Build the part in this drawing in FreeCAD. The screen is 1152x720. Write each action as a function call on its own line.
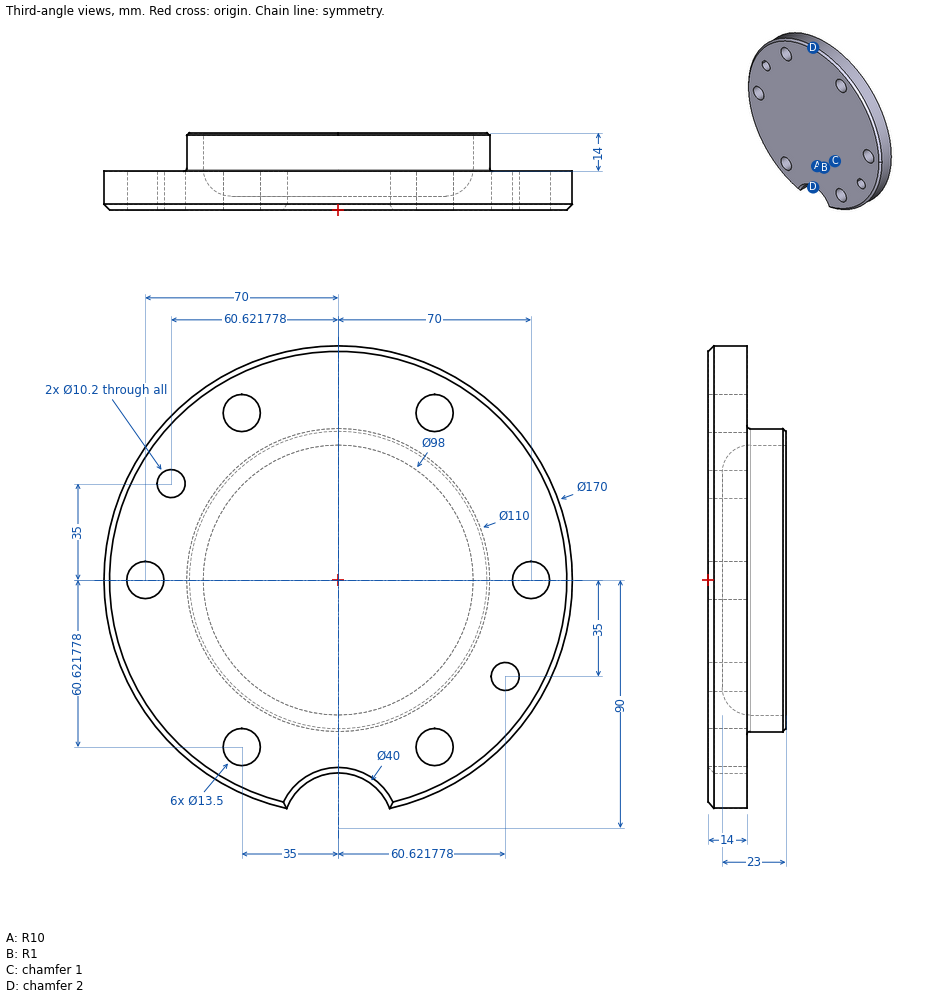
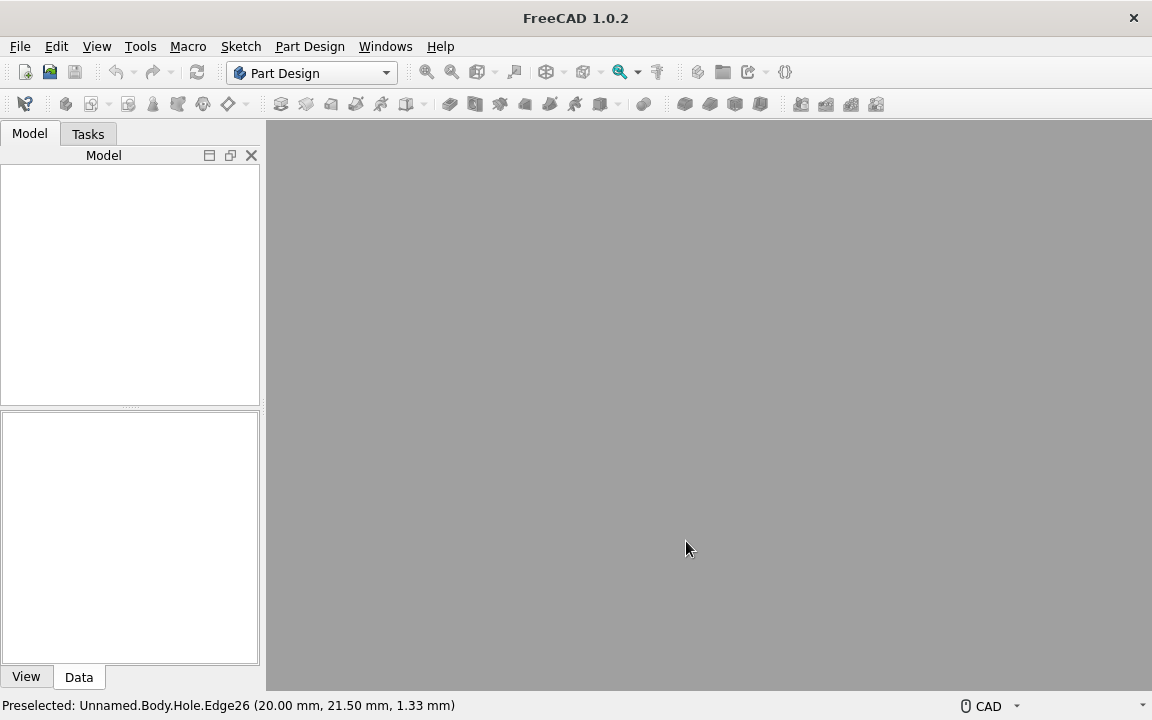
click(25, 72)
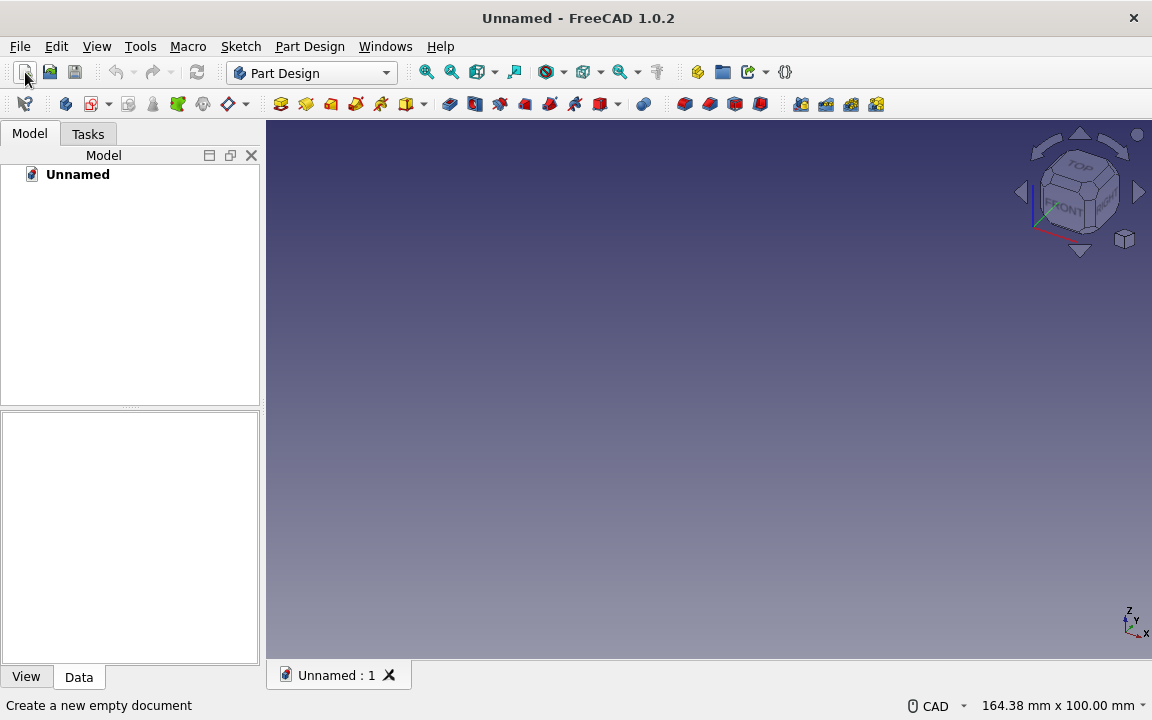
click(90, 104)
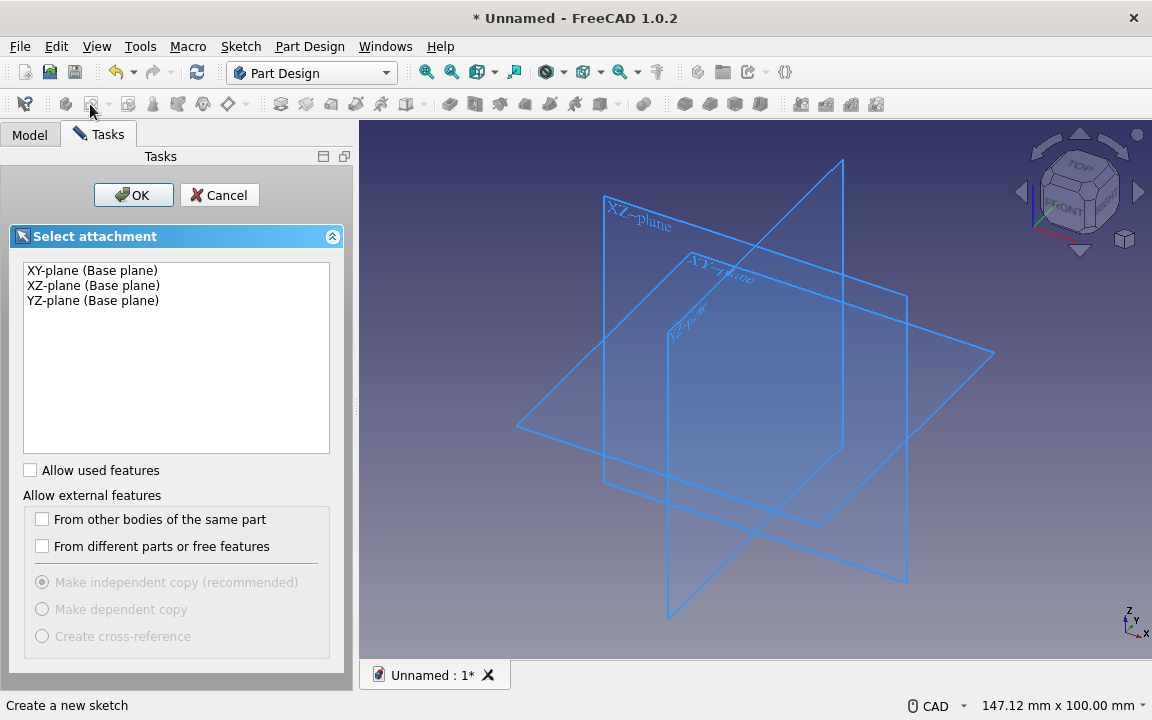
click(84, 286)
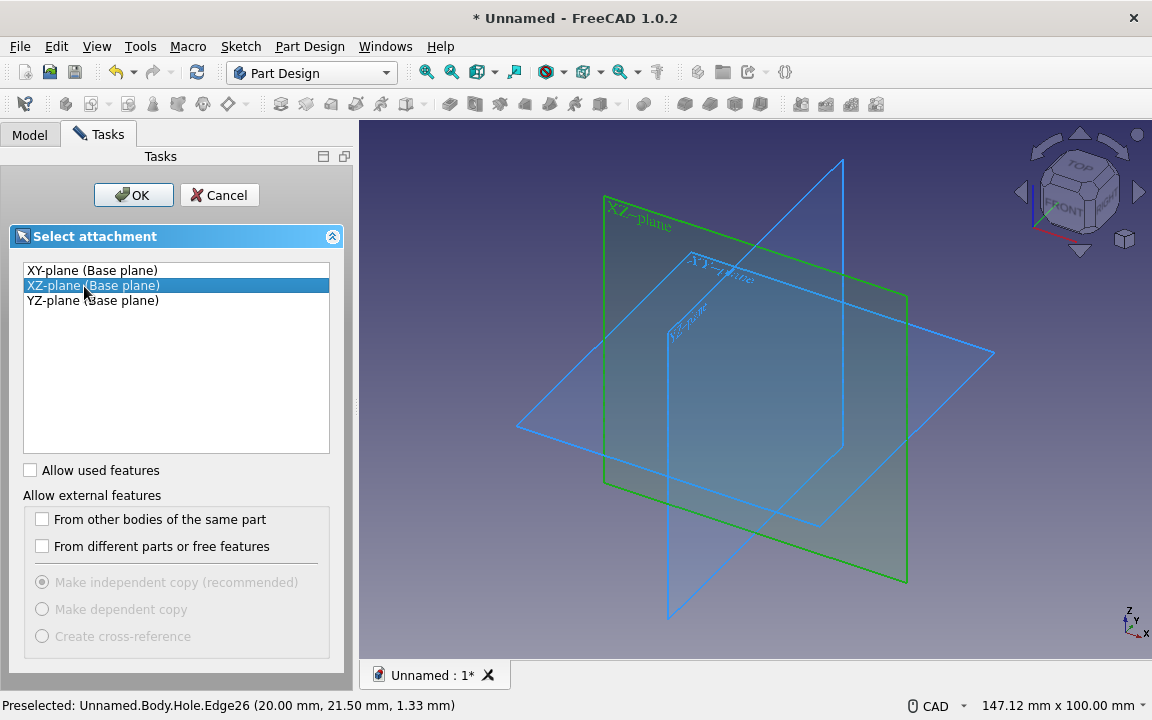
click(134, 195)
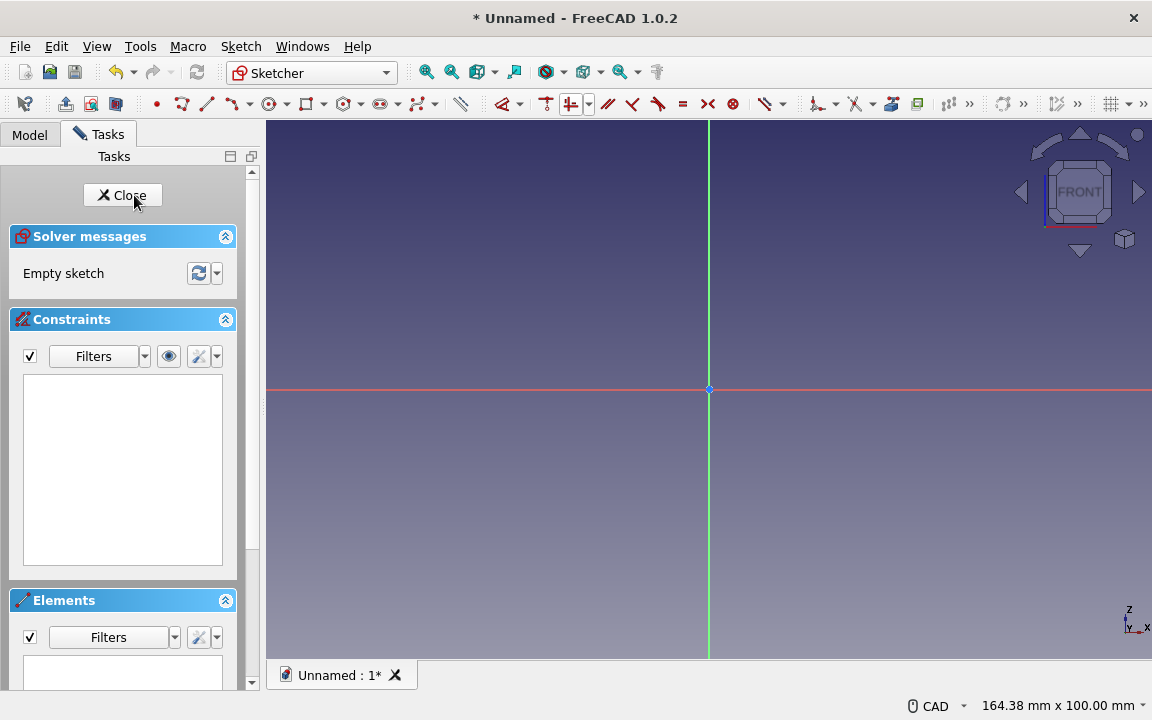
scroll(601, 390, down, 5)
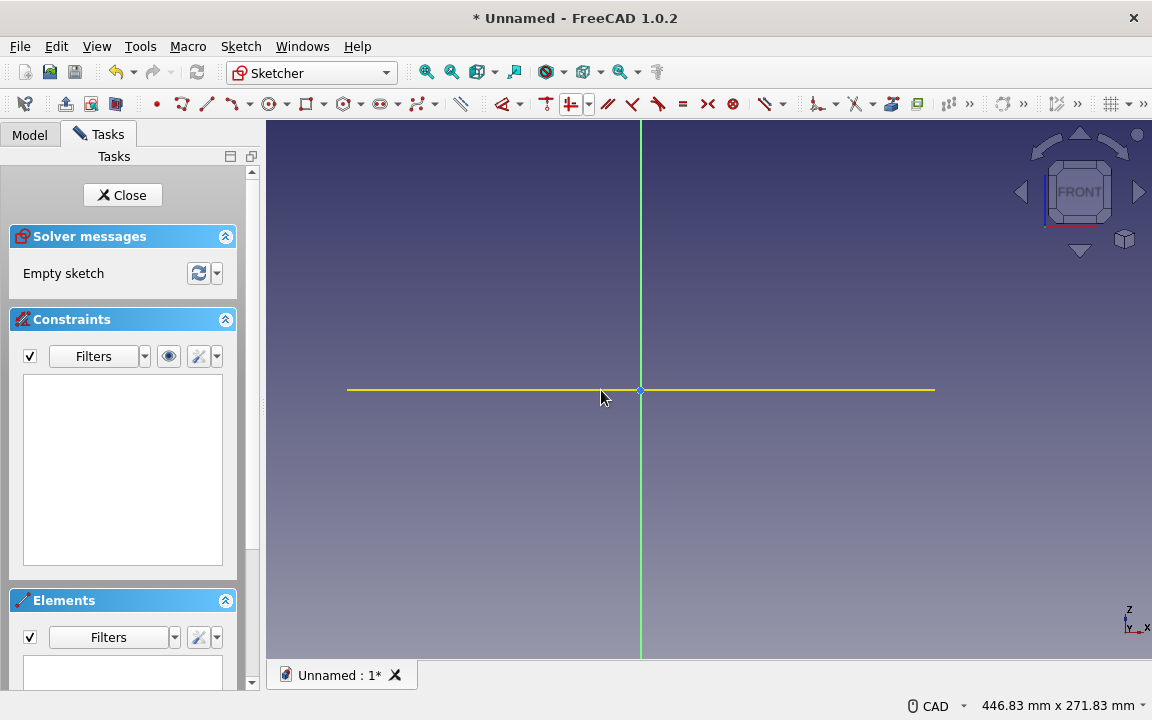
click(268, 104)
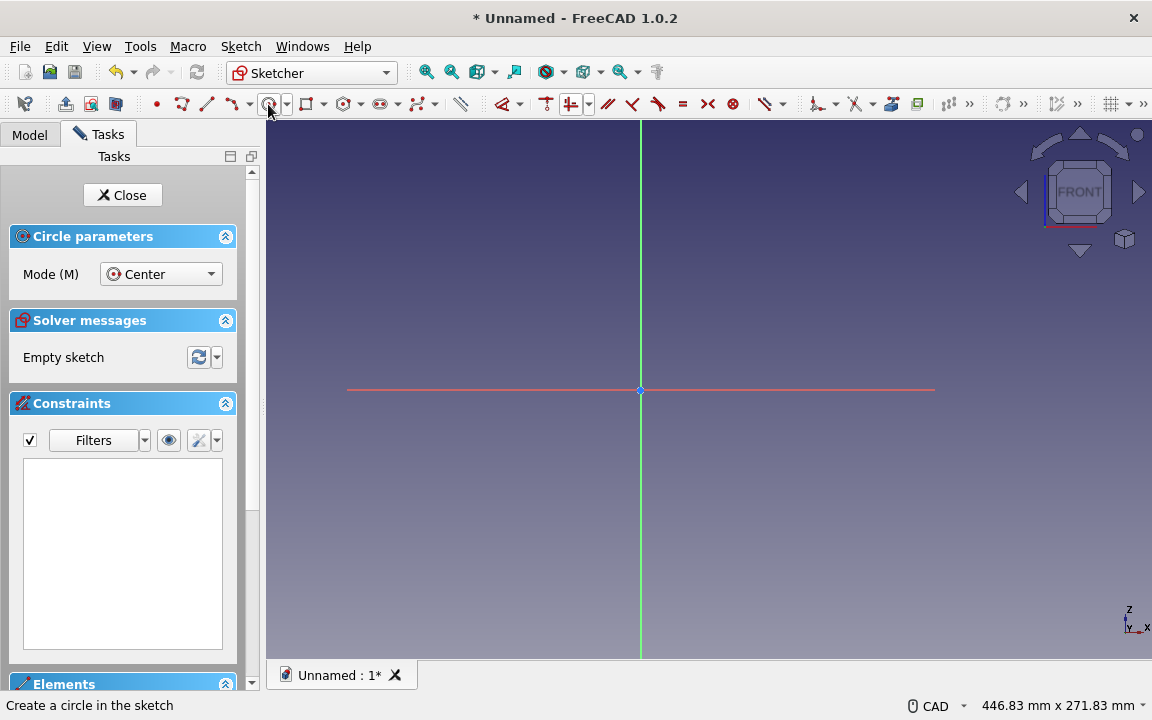
click(641, 390)
click(760, 271)
key(Escape)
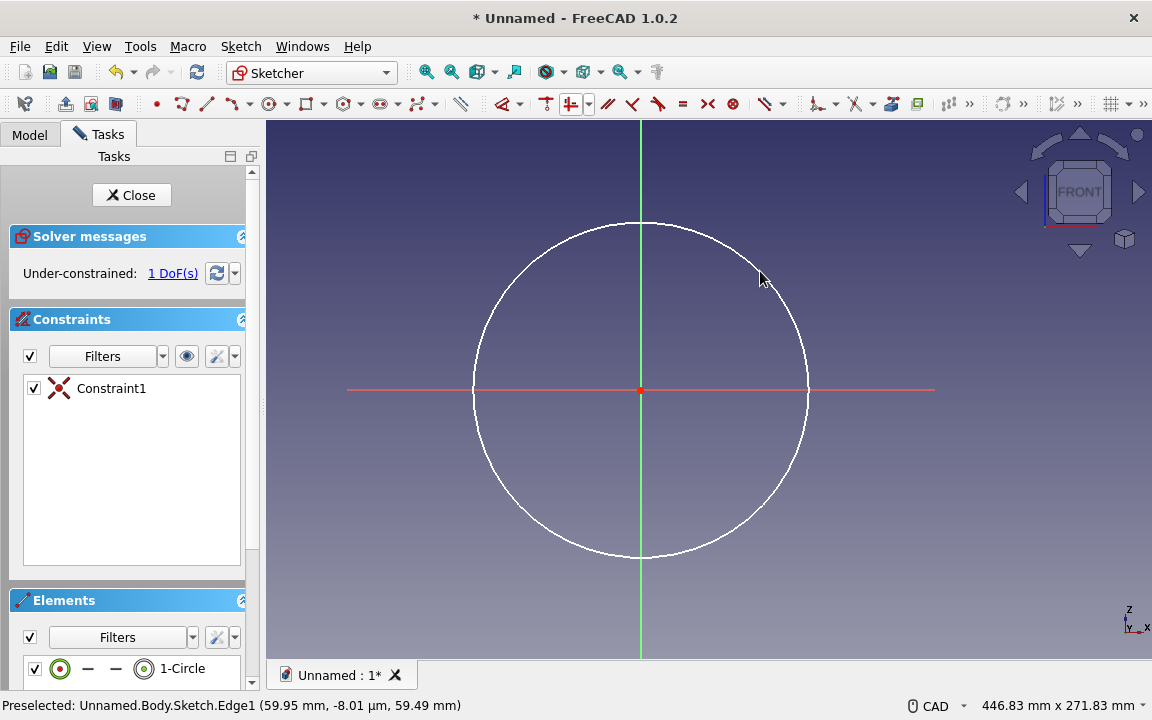
click(759, 271)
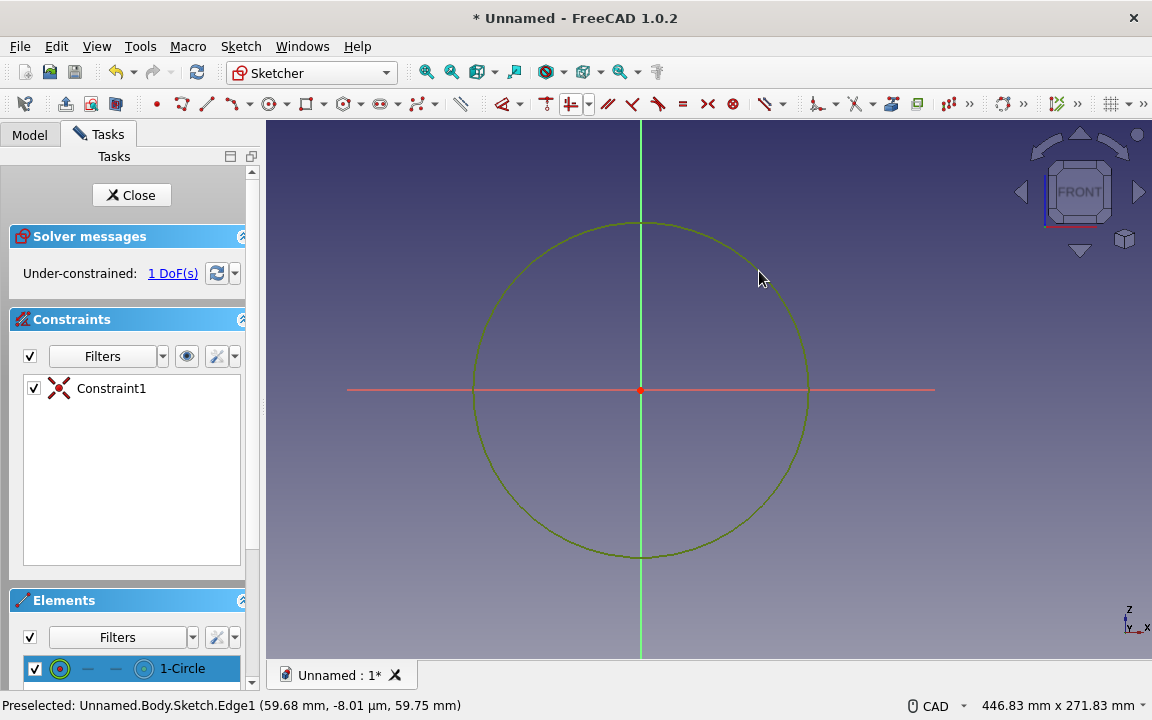
key(k)
key(o)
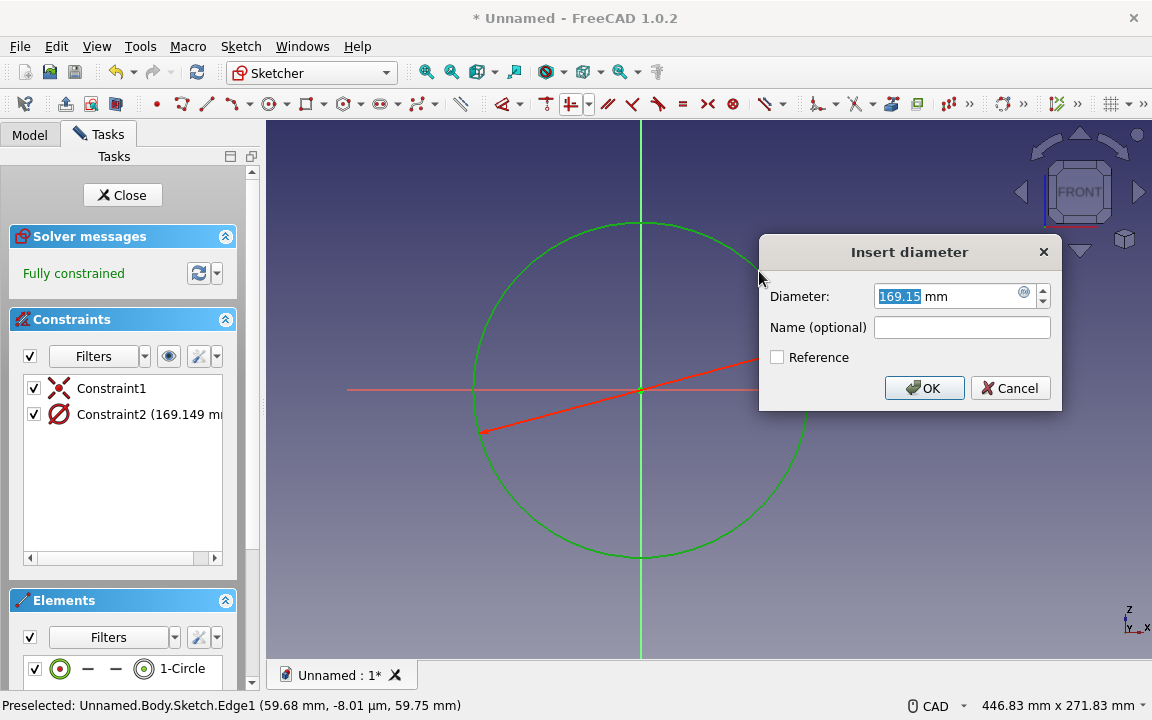
text(170)
key(Return)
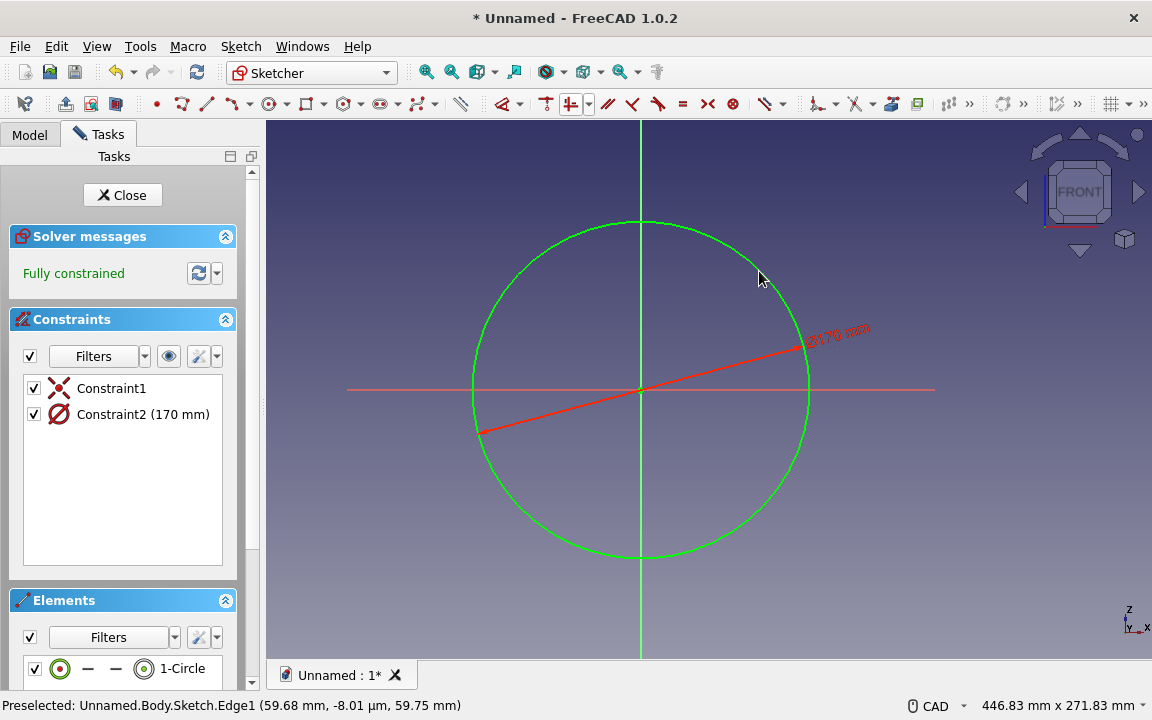
click(123, 195)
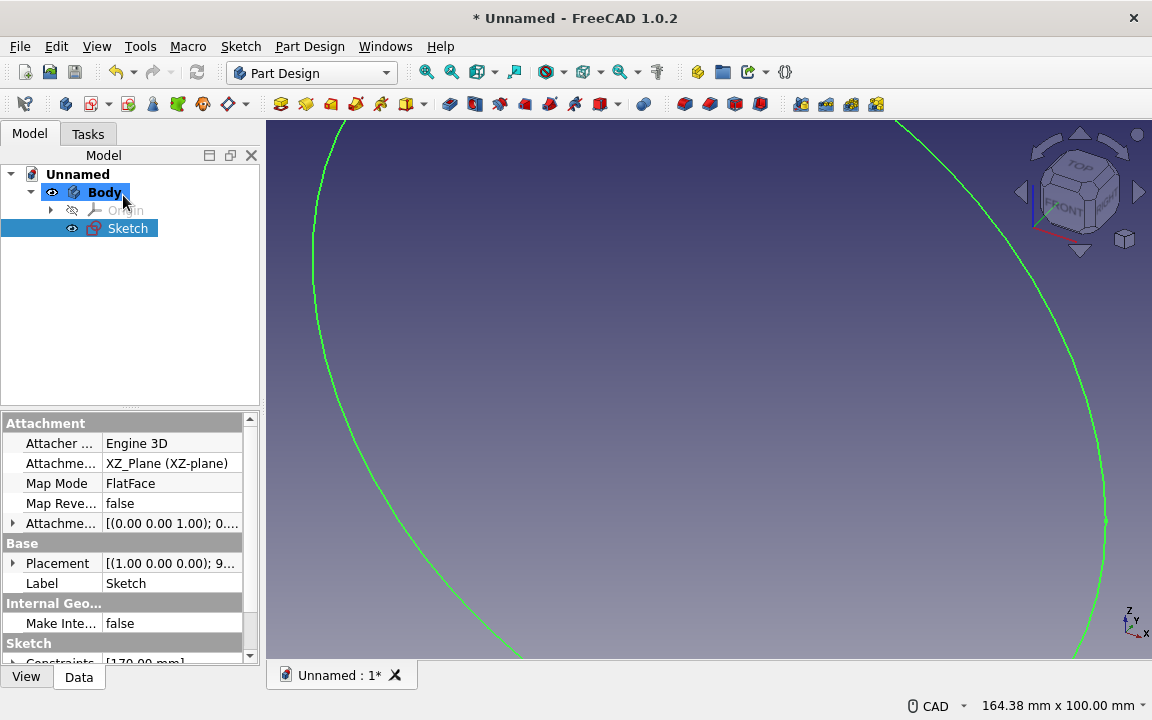
click(281, 104)